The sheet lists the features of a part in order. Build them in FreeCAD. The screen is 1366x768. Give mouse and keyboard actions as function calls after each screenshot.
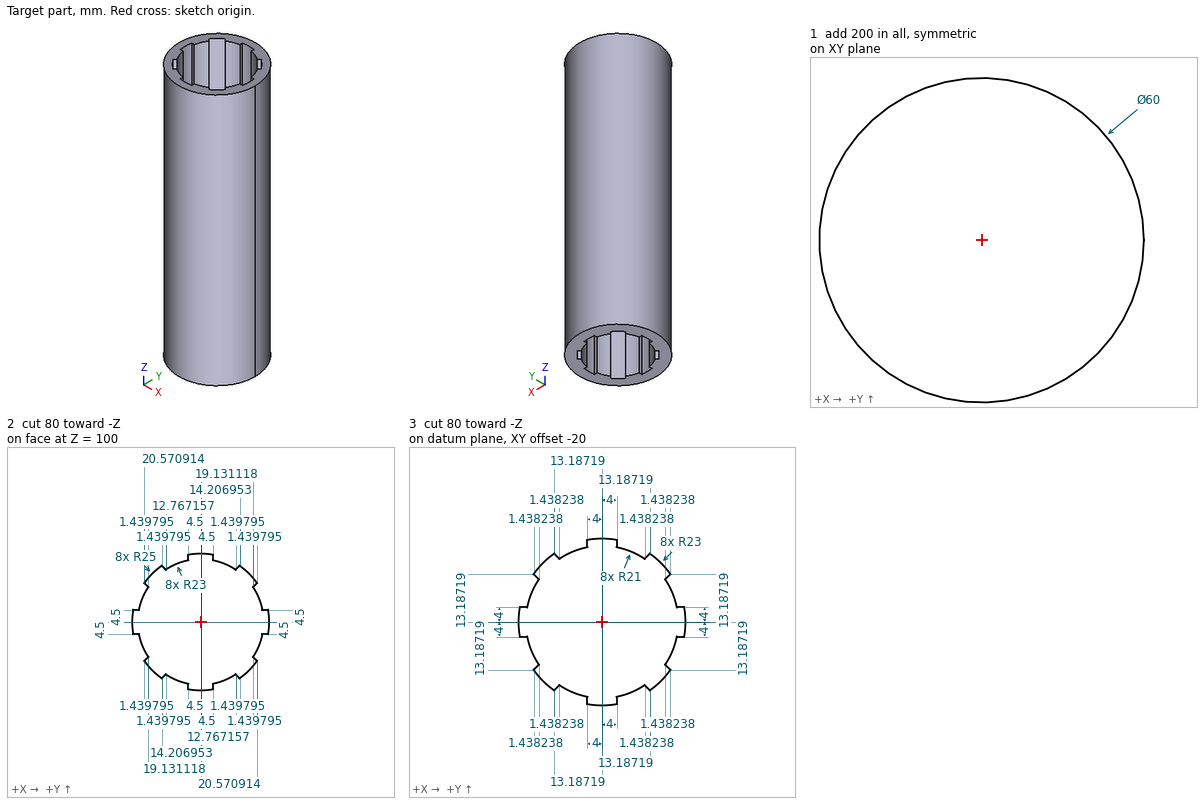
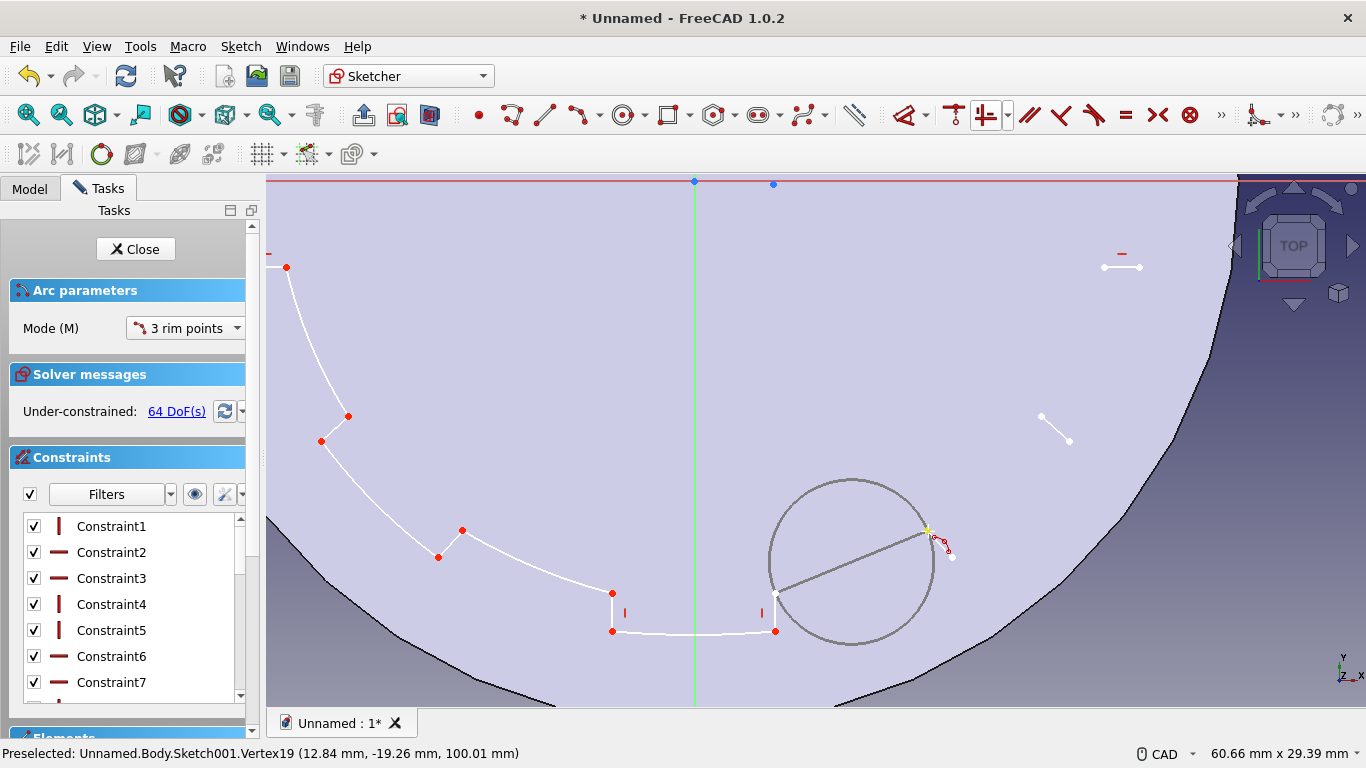
scroll(854, 567, up, 4)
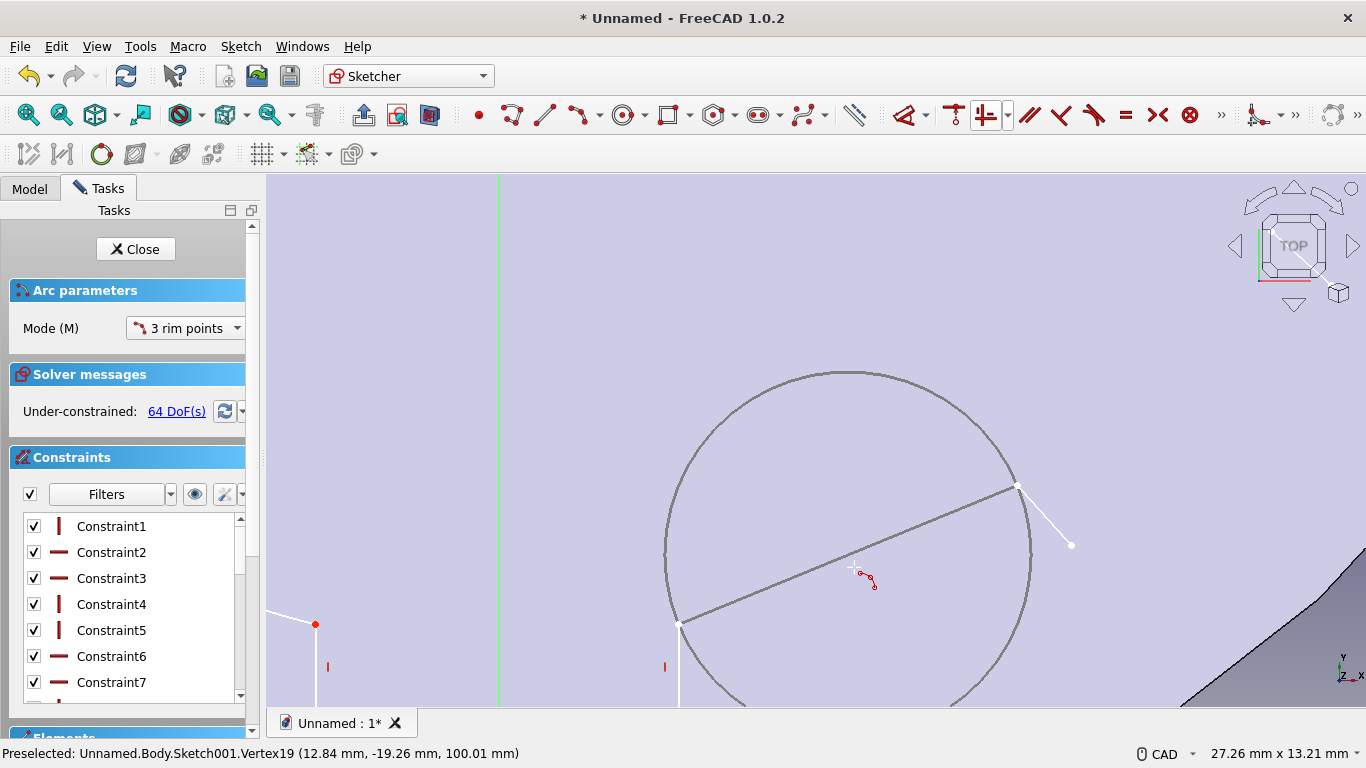
click(854, 566)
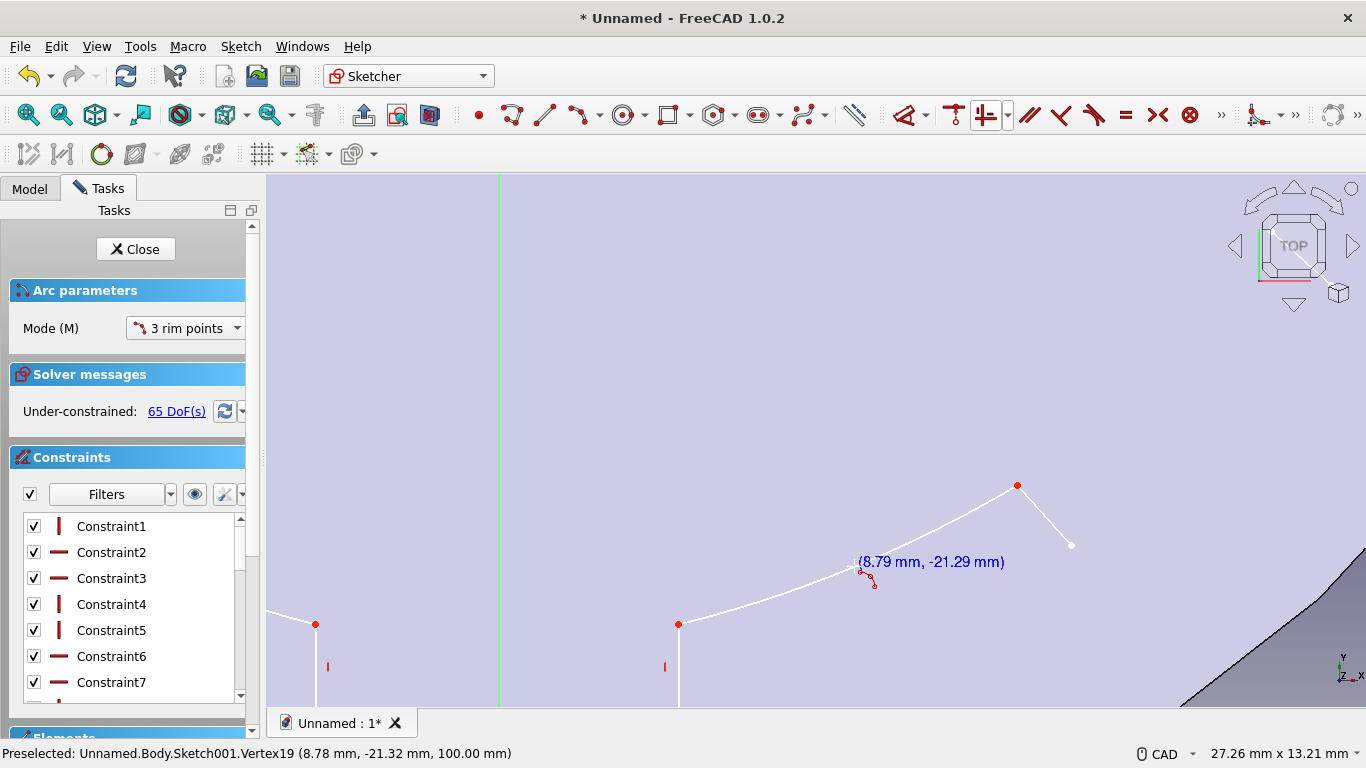
click(1072, 546)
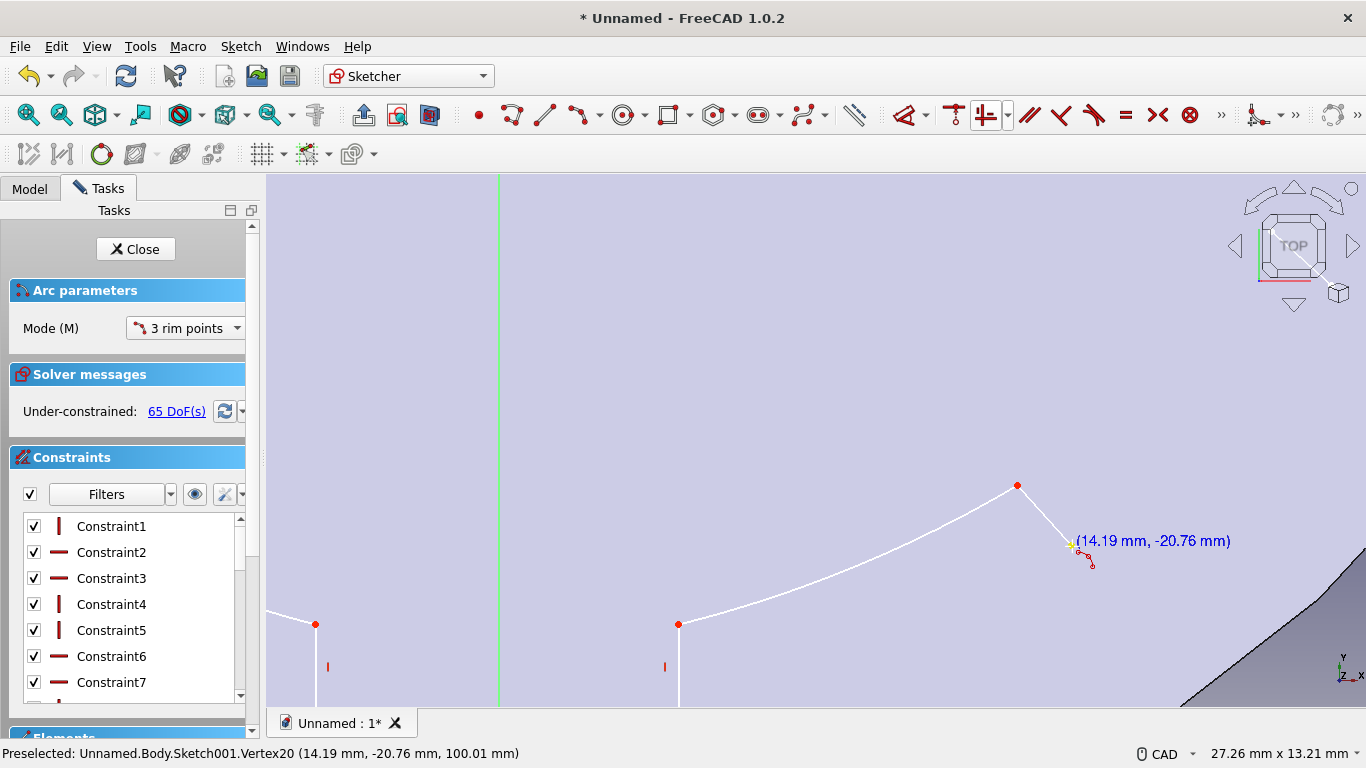
scroll(797, 586, down, 9)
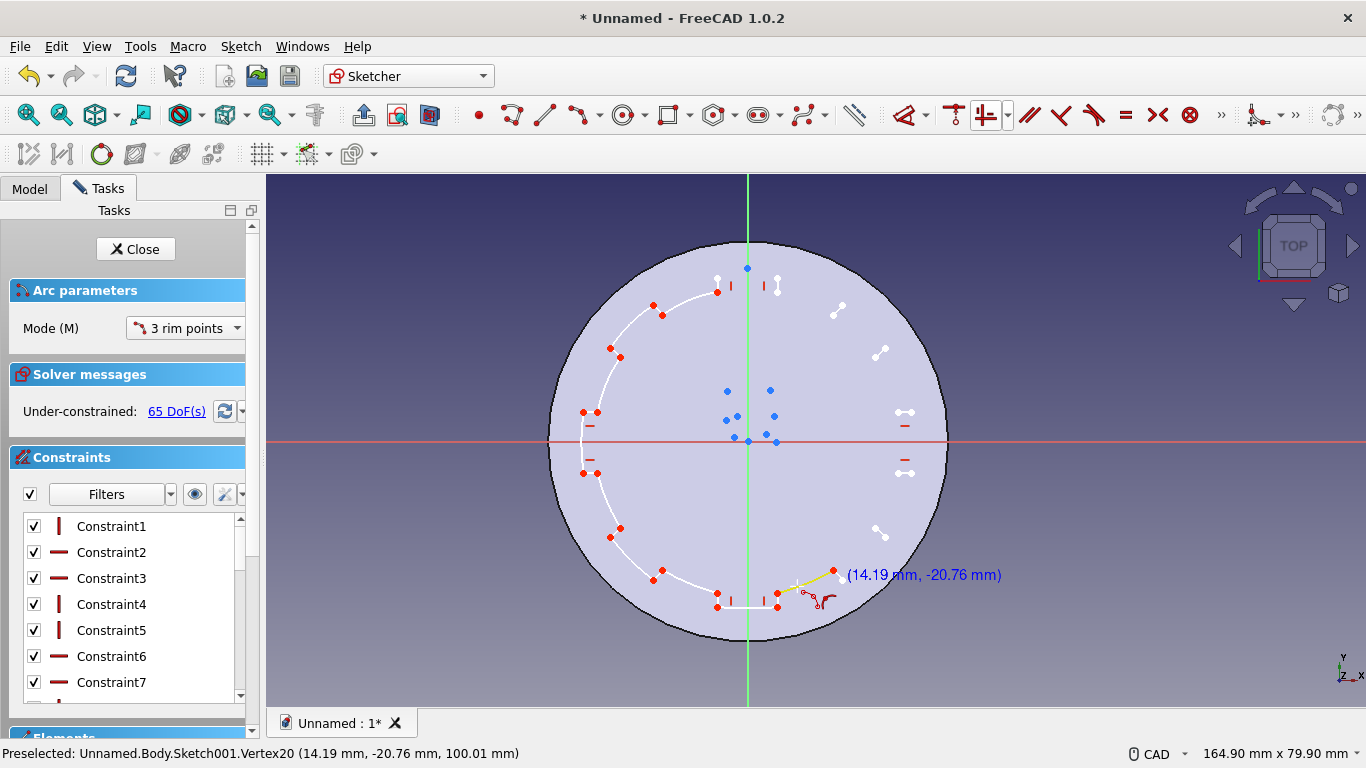
scroll(885, 536, up, 5)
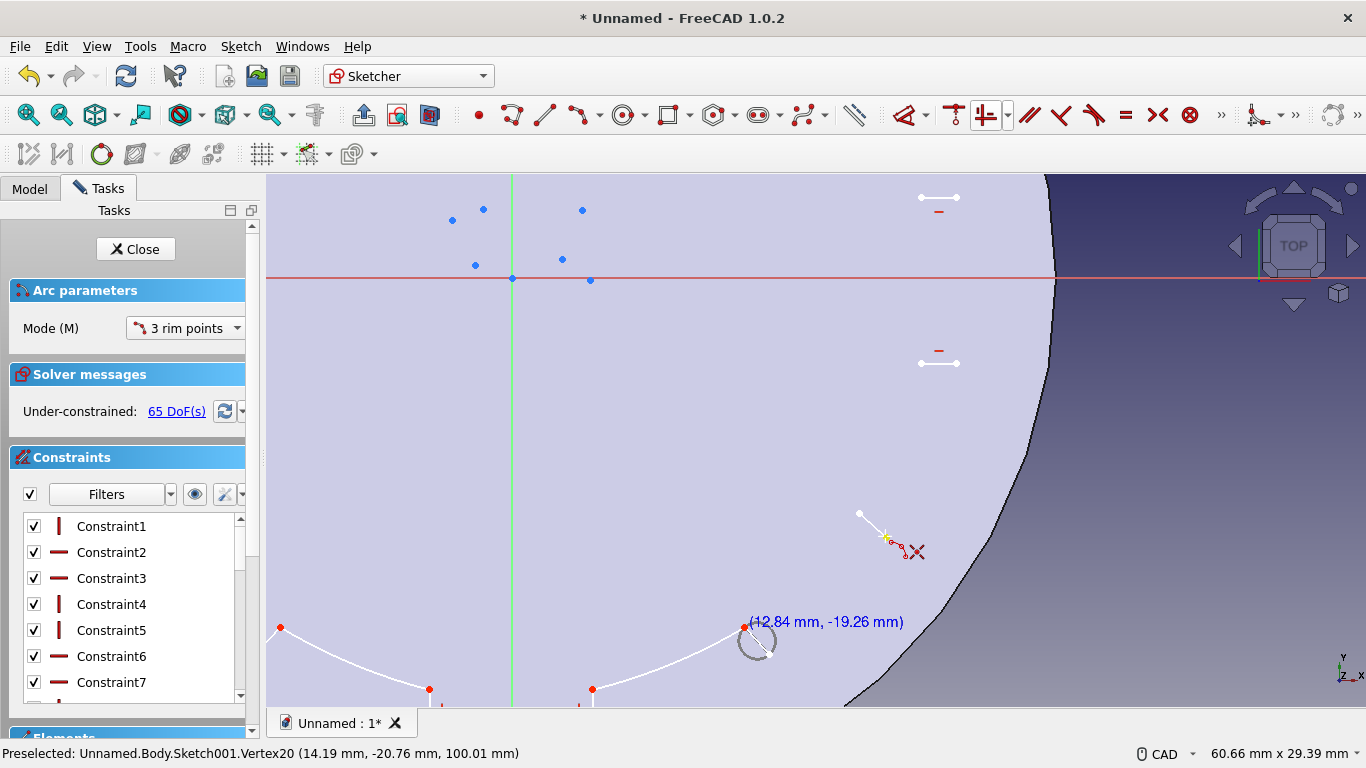
click(886, 538)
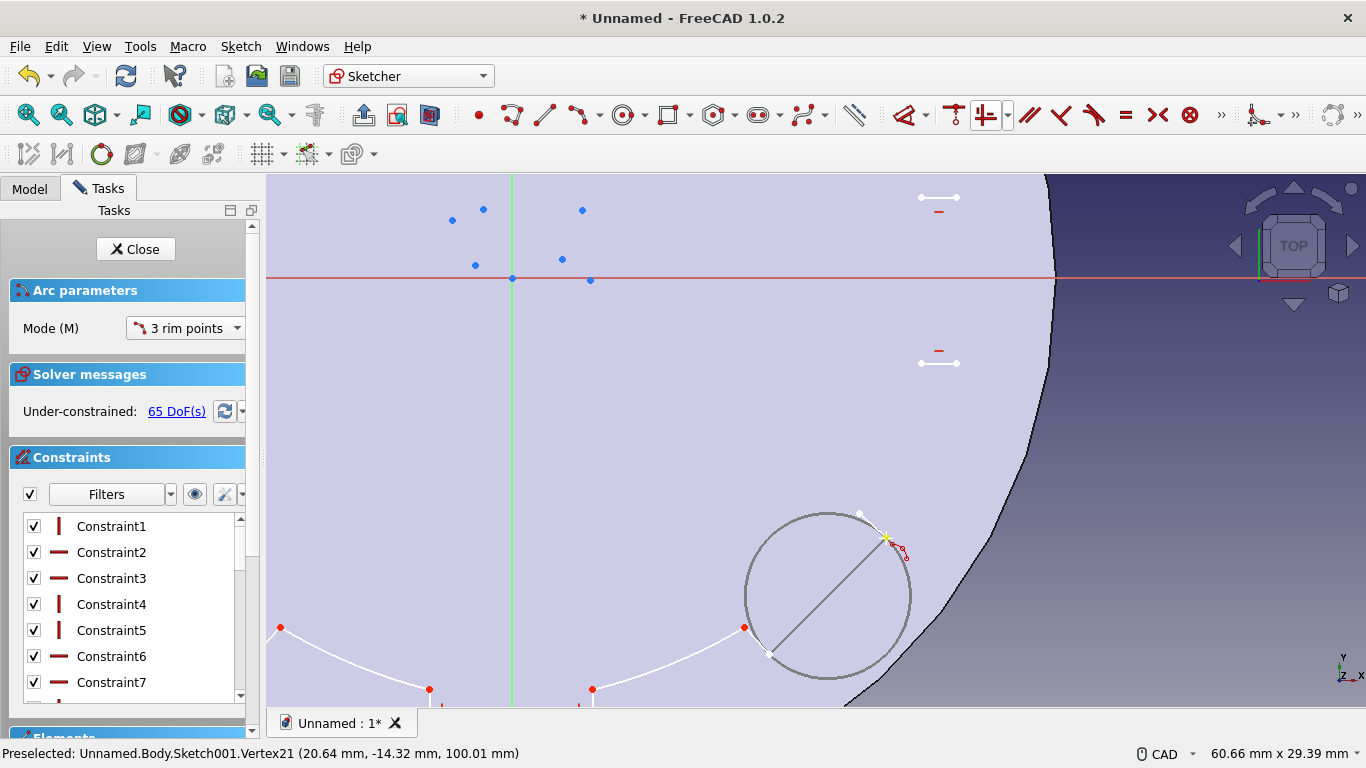
scroll(833, 599, up, 4)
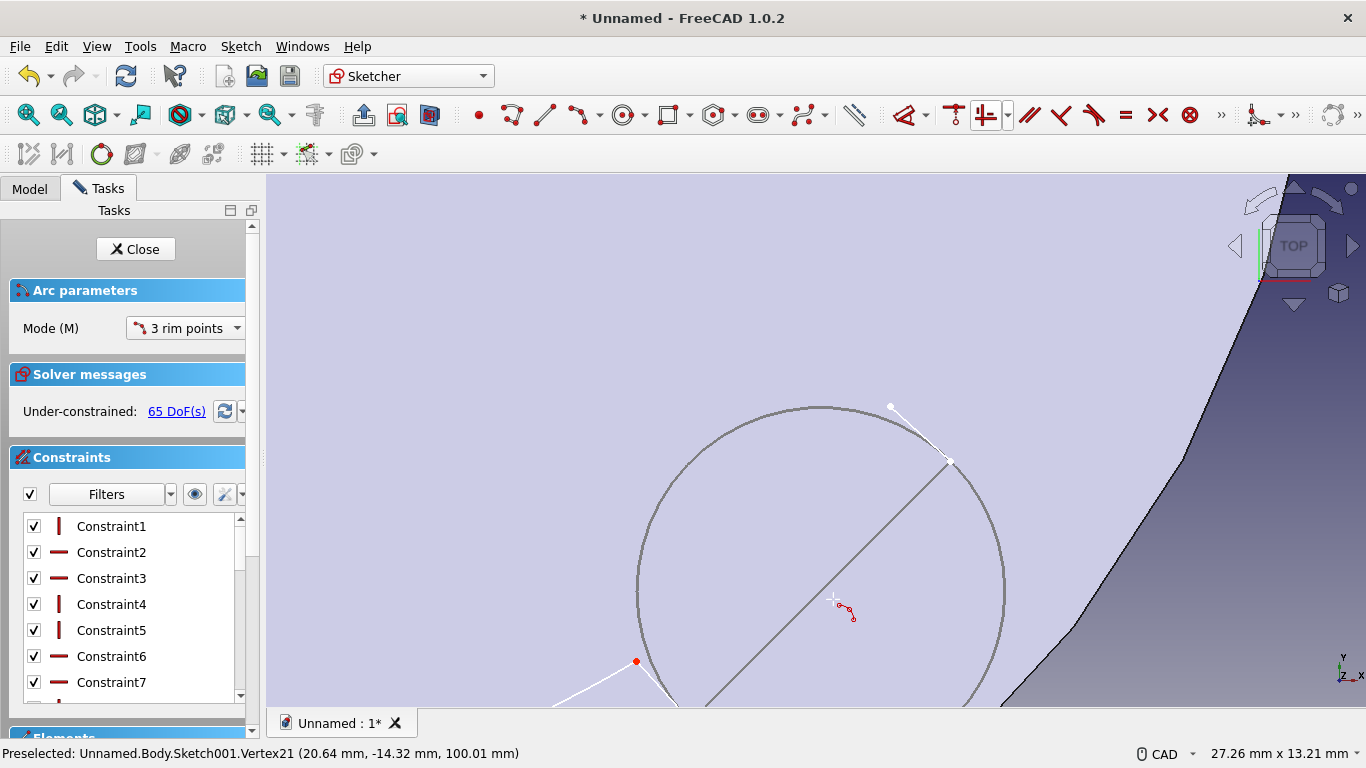
click(832, 597)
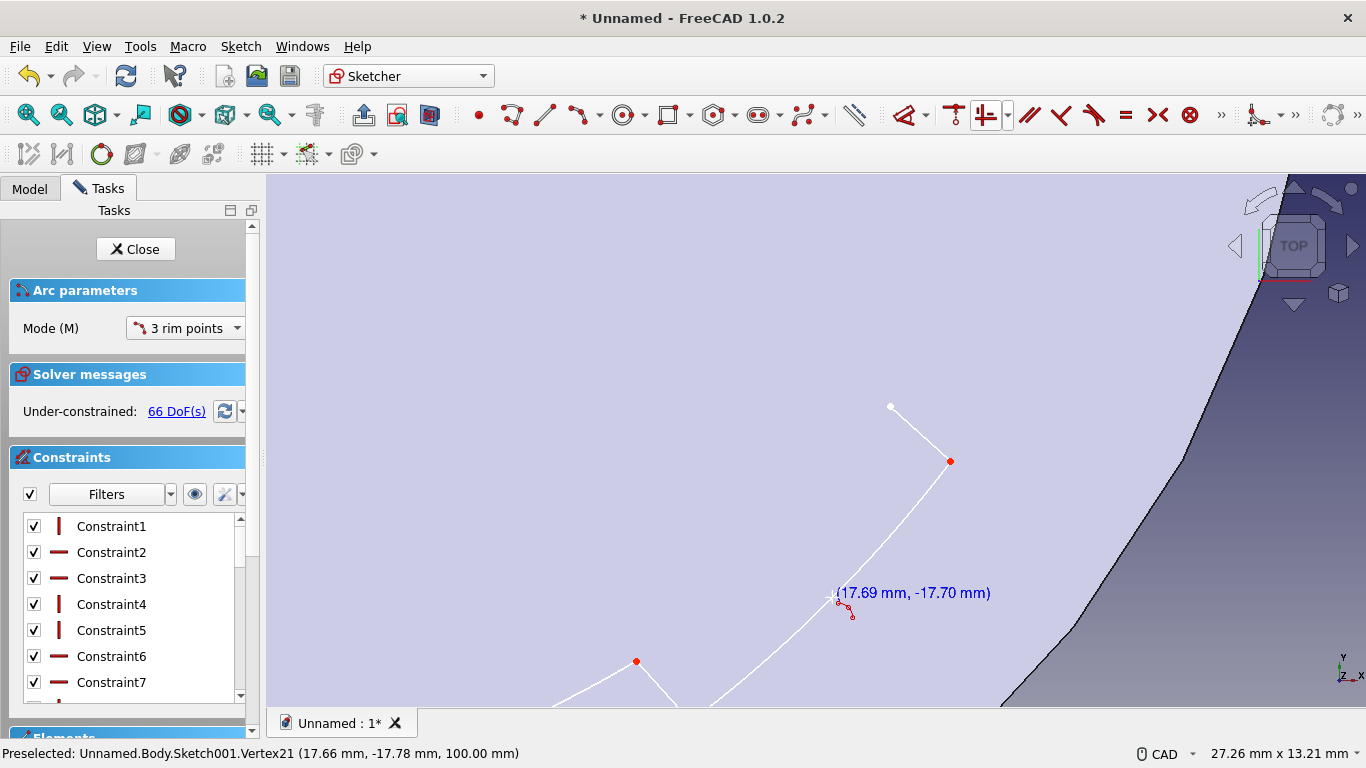
click(890, 407)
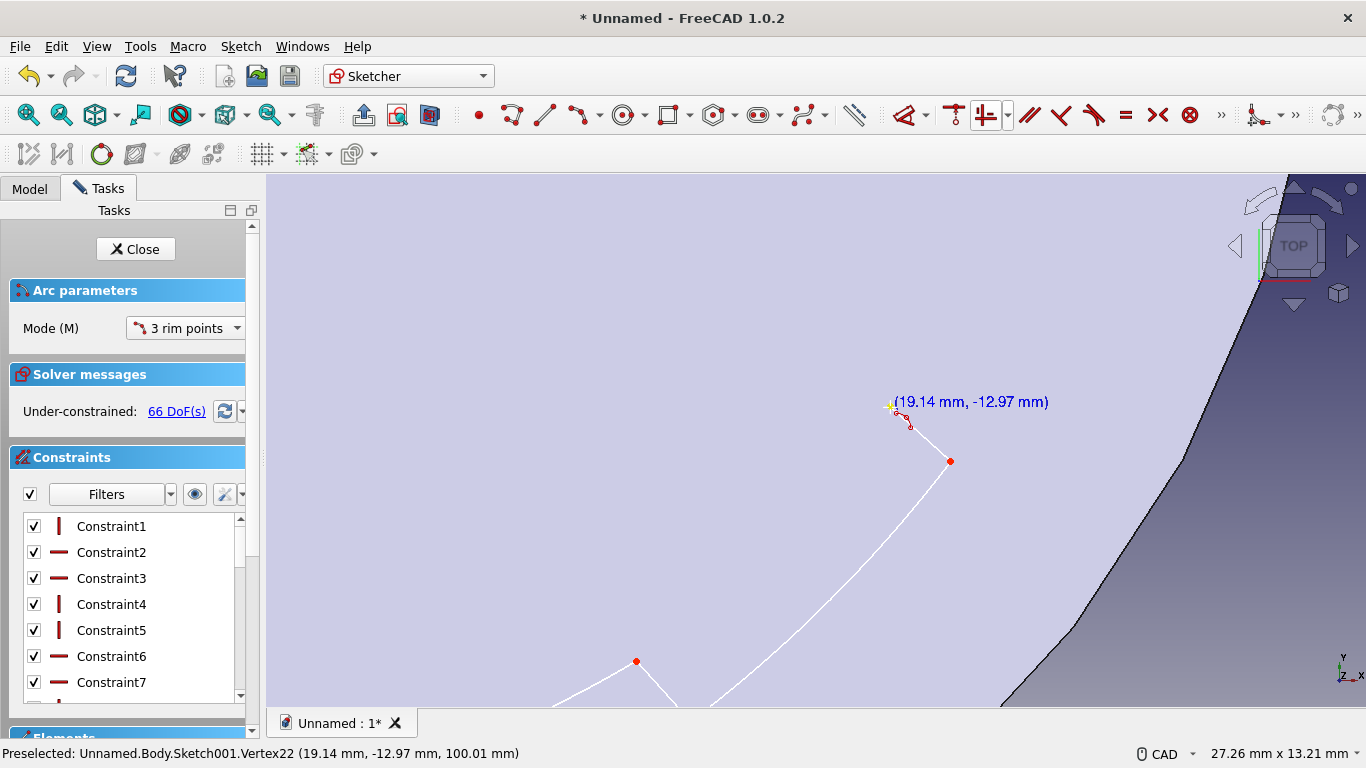
scroll(872, 551, down, 9)